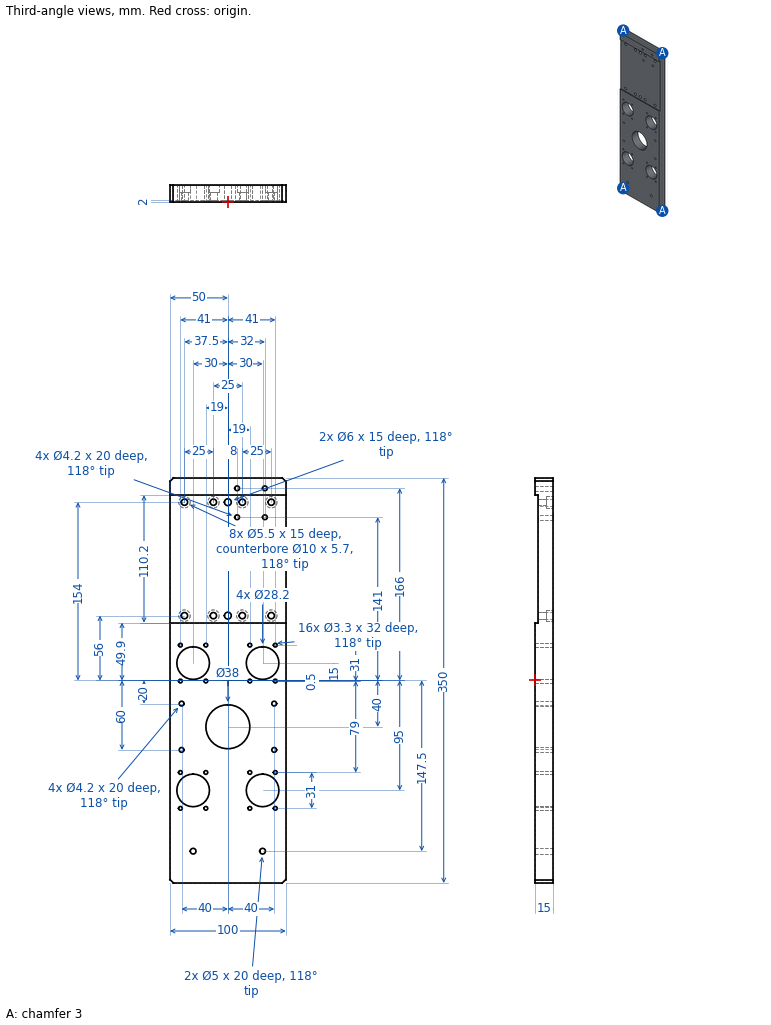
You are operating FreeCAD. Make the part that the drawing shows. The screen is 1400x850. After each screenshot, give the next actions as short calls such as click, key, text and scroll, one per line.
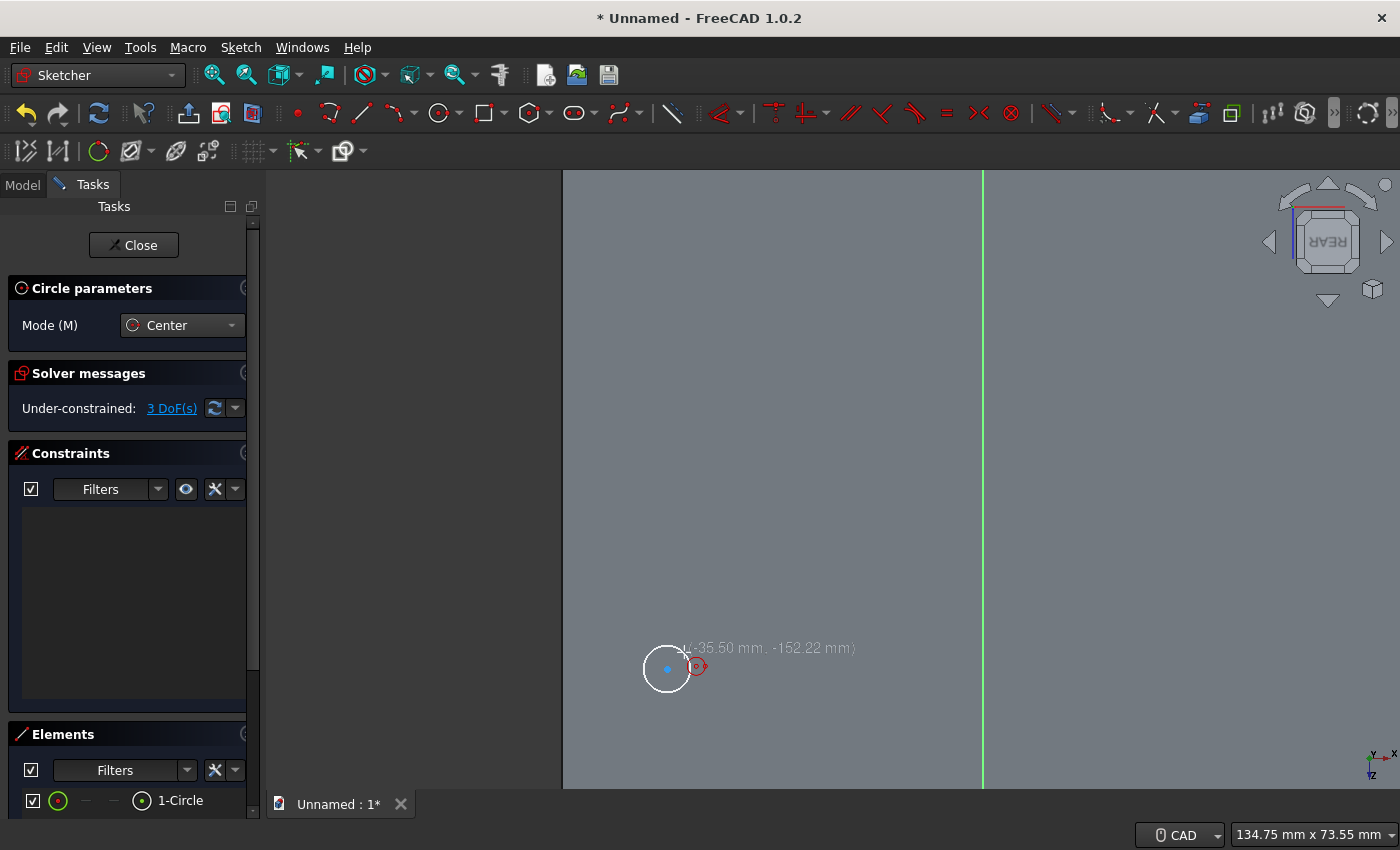
click(878, 668)
click(894, 652)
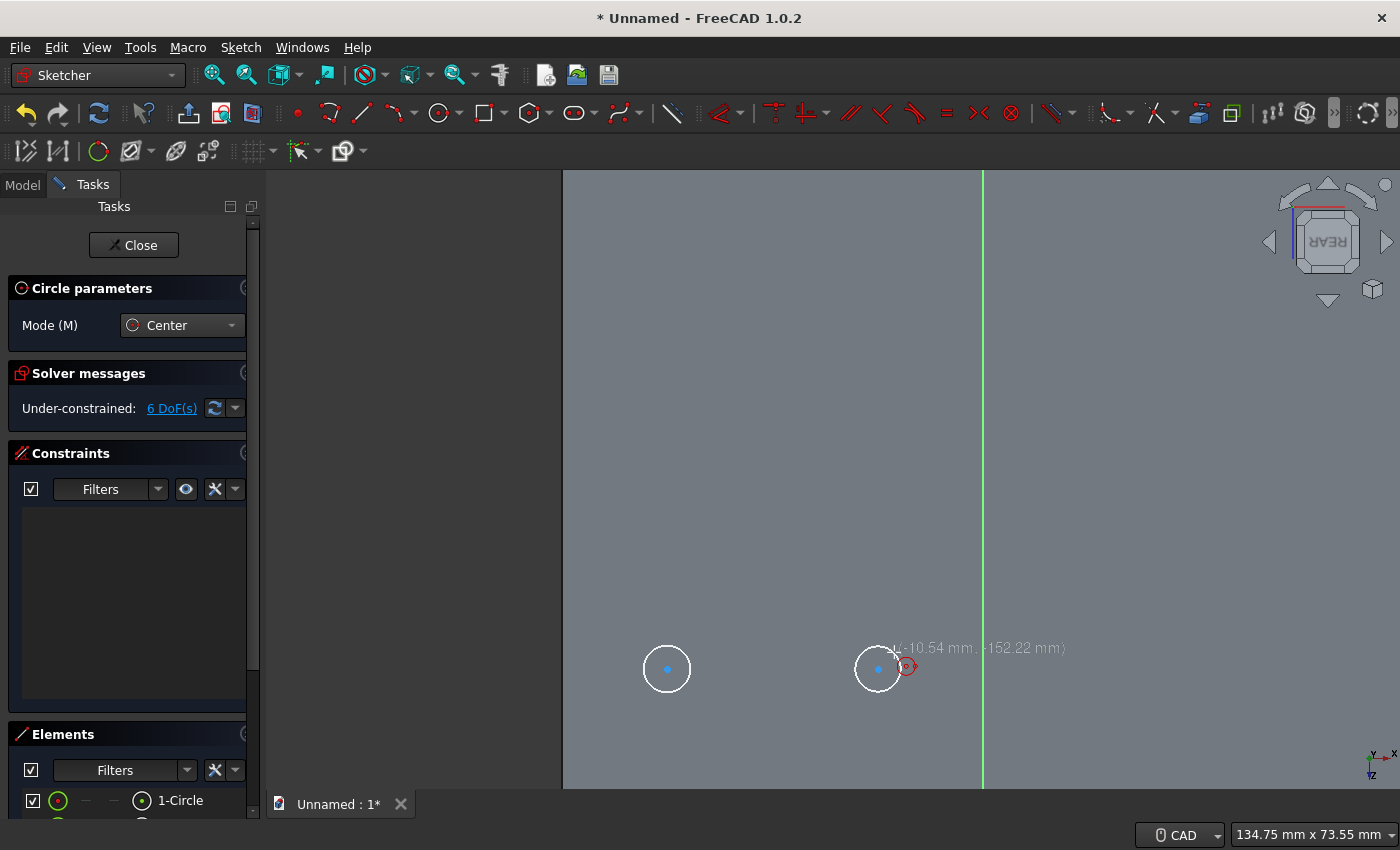
click(1088, 668)
click(1104, 652)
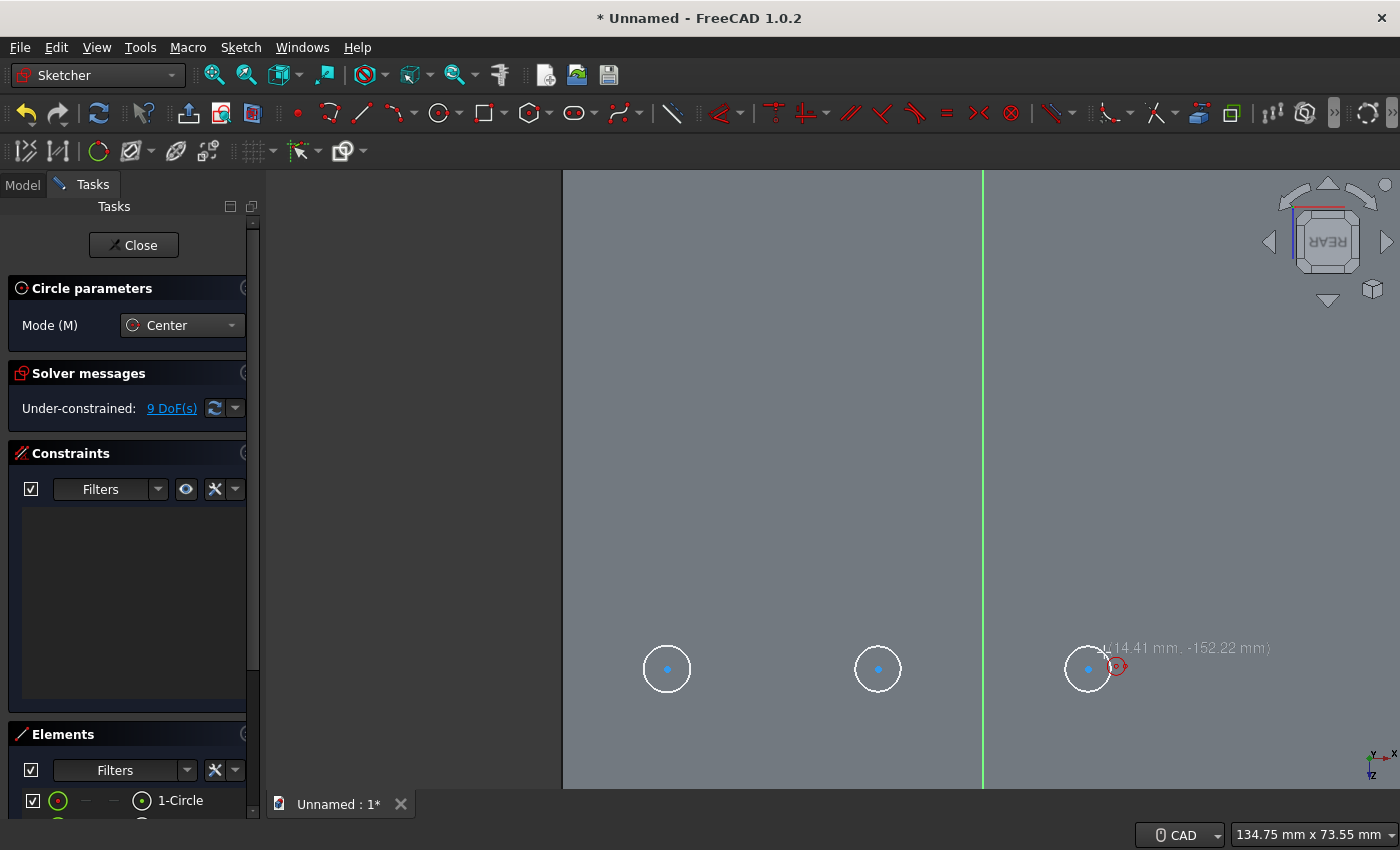
scroll(670, 673, down, 6)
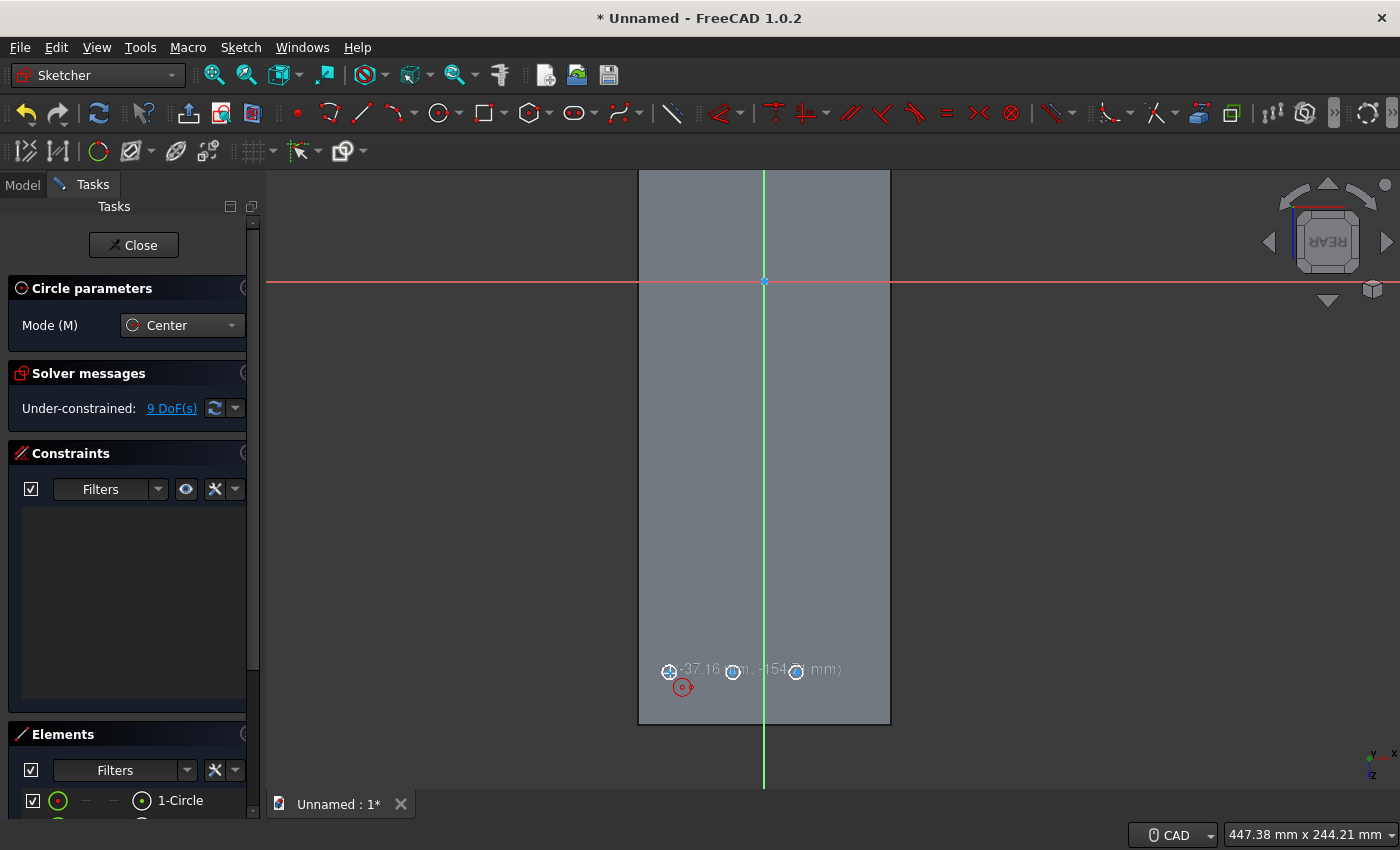
scroll(859, 672, up, 6)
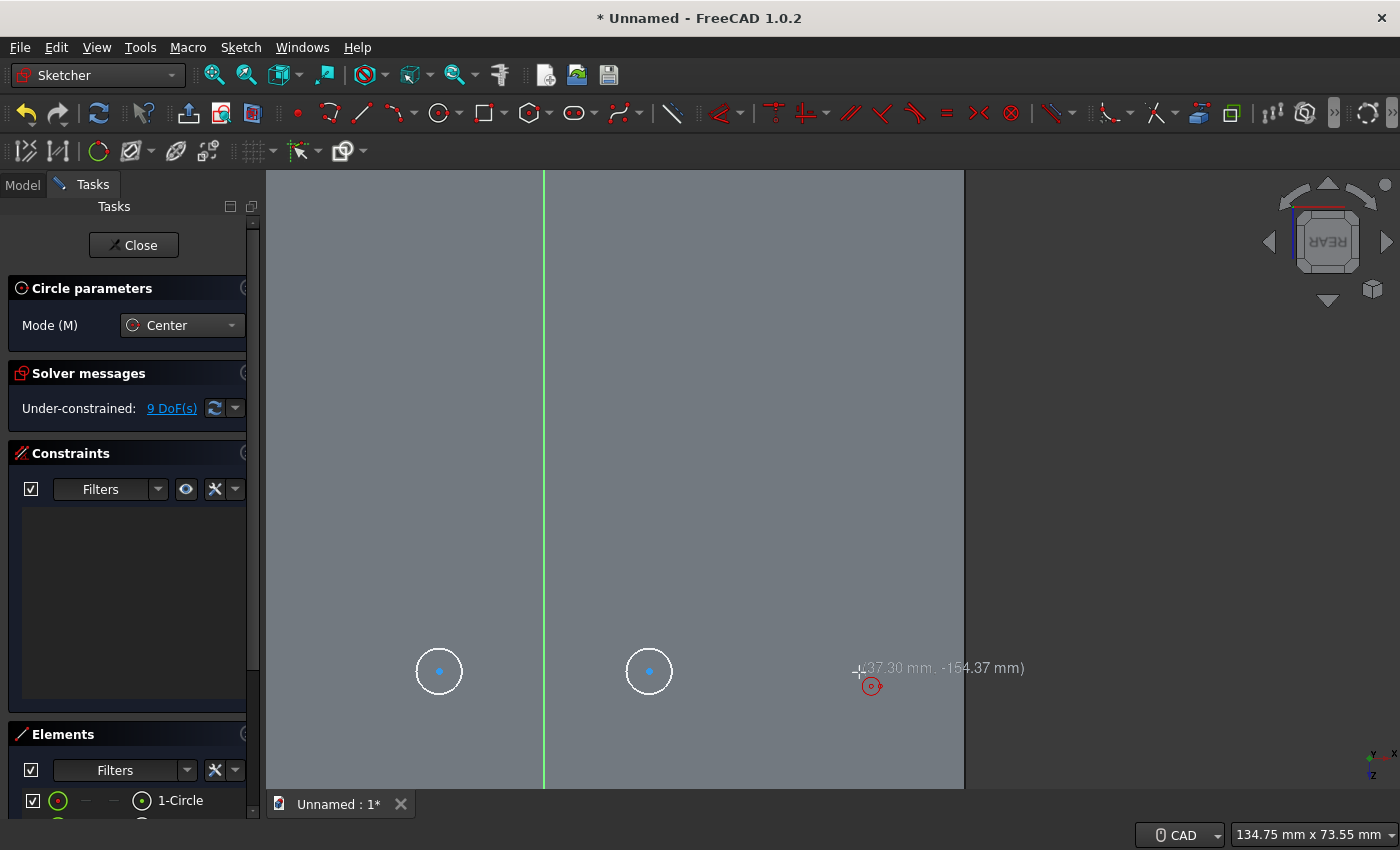
click(859, 670)
click(876, 654)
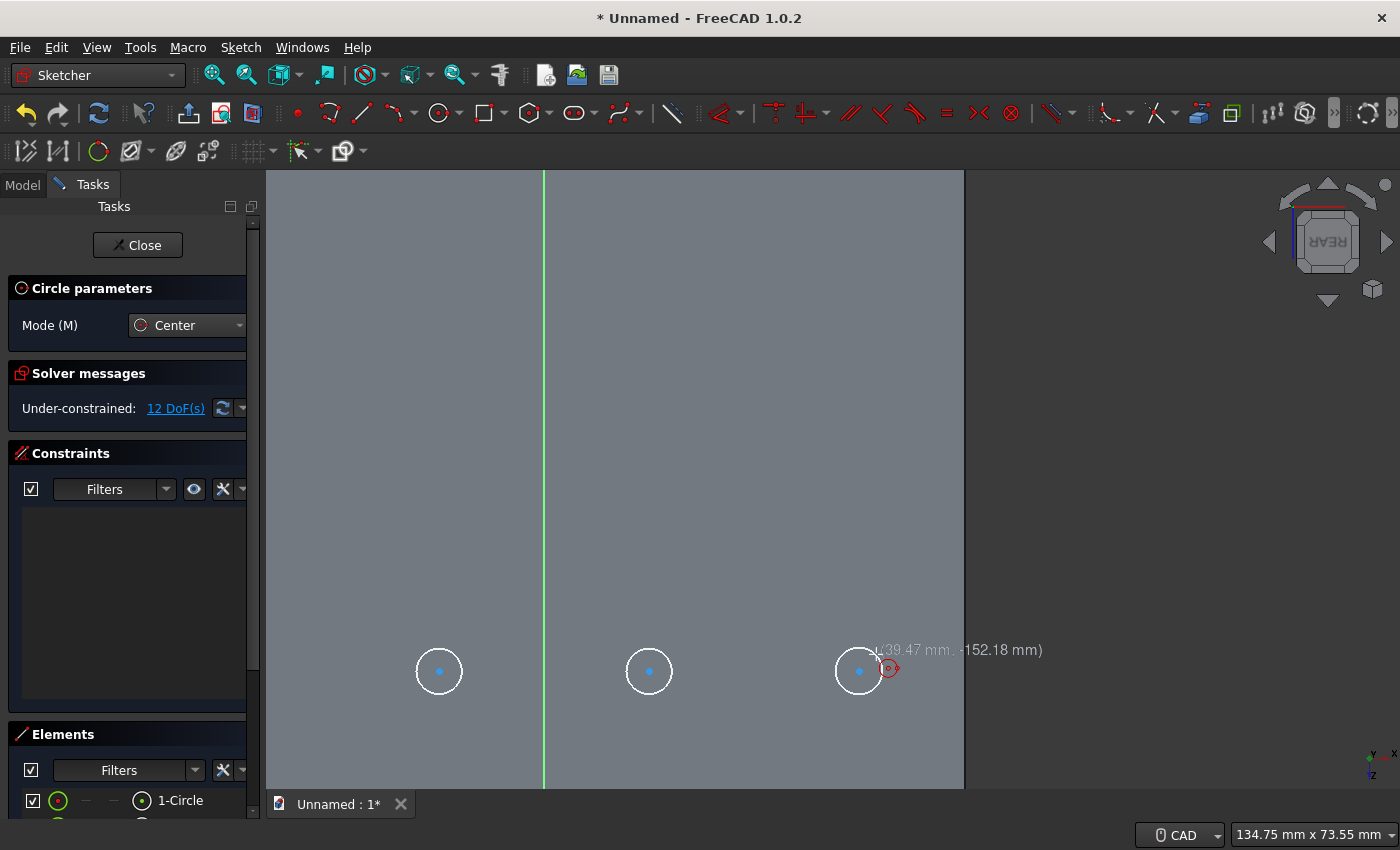
scroll(860, 672, down, 6)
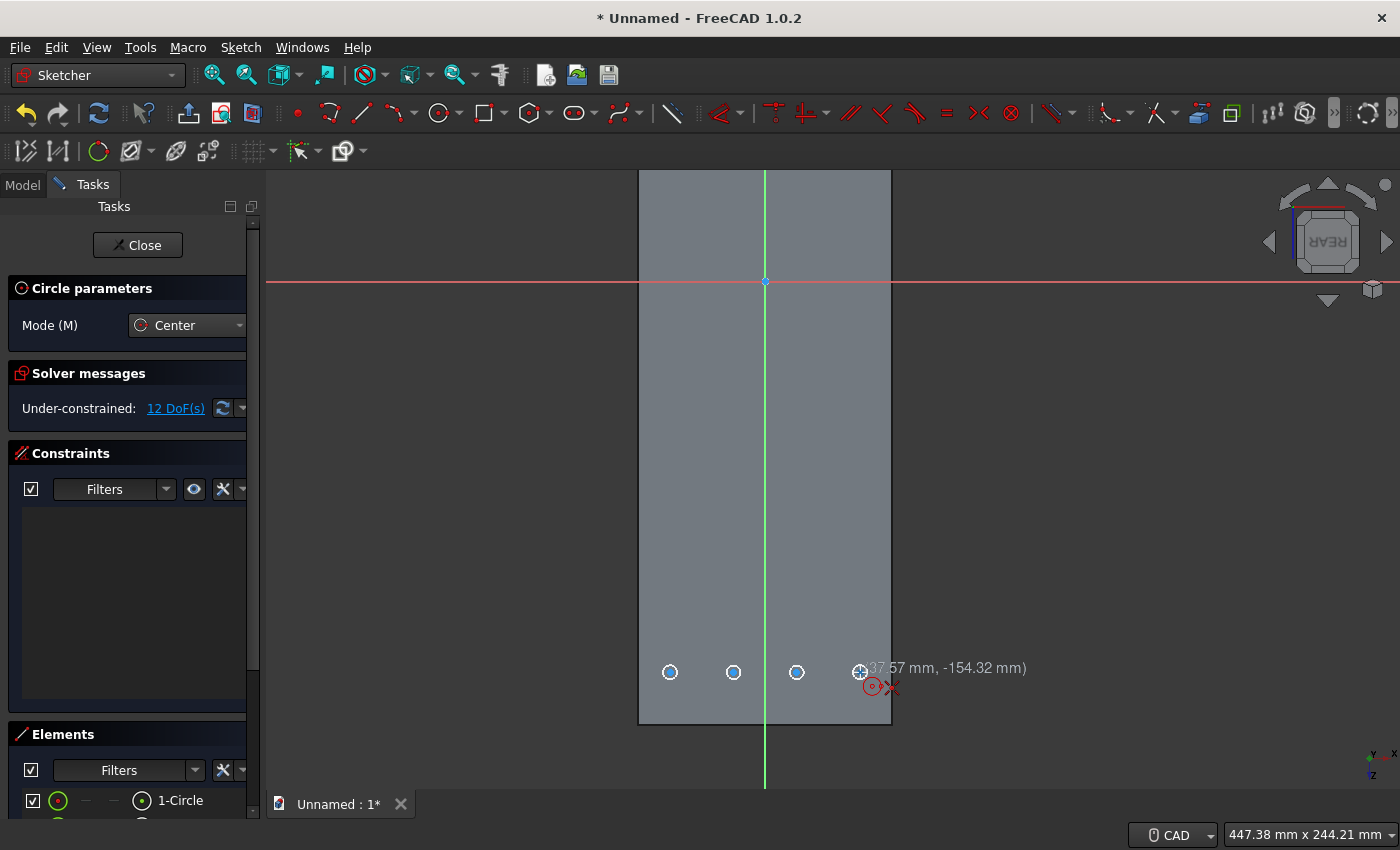
scroll(670, 424, up, 6)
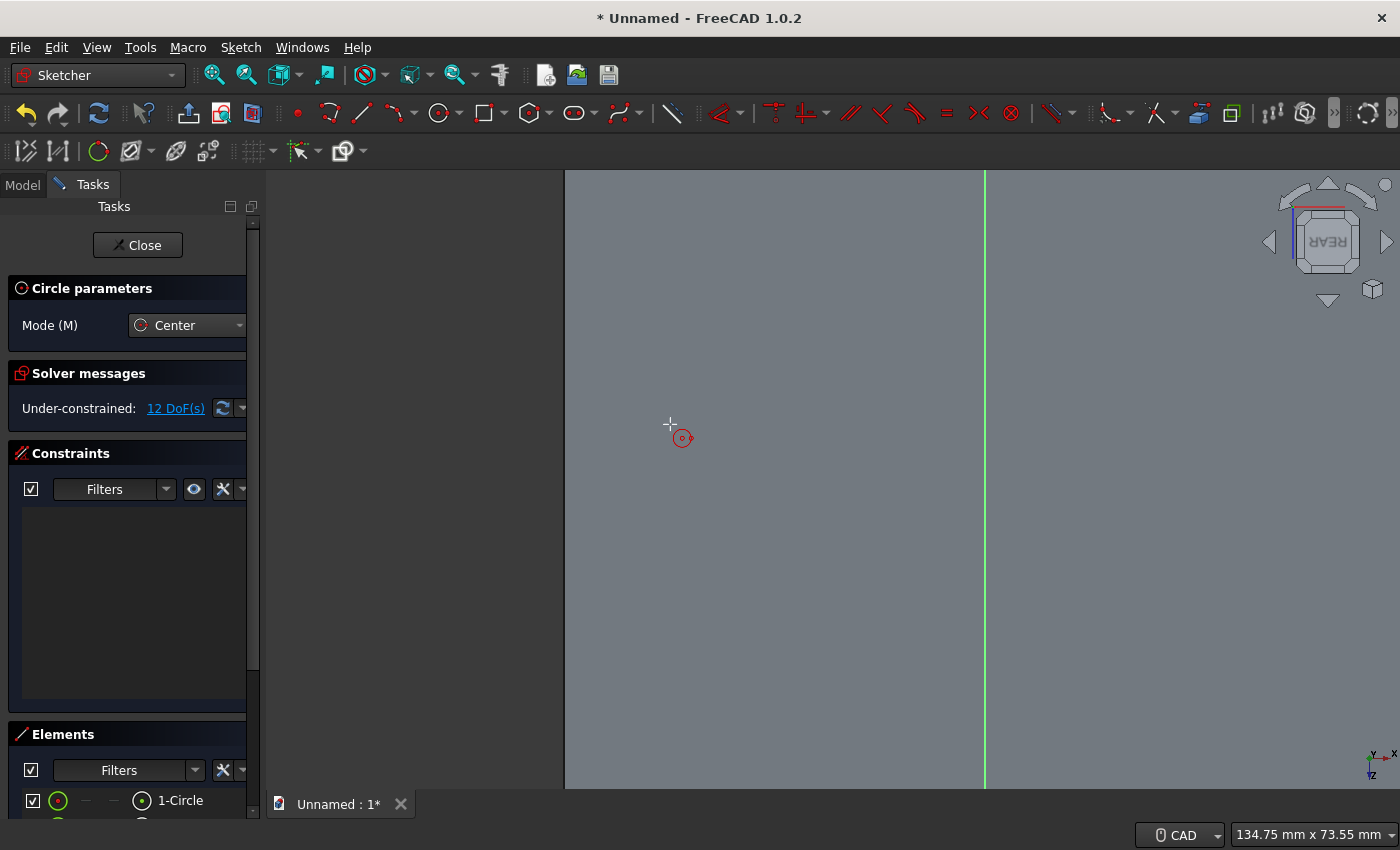
click(669, 422)
click(686, 406)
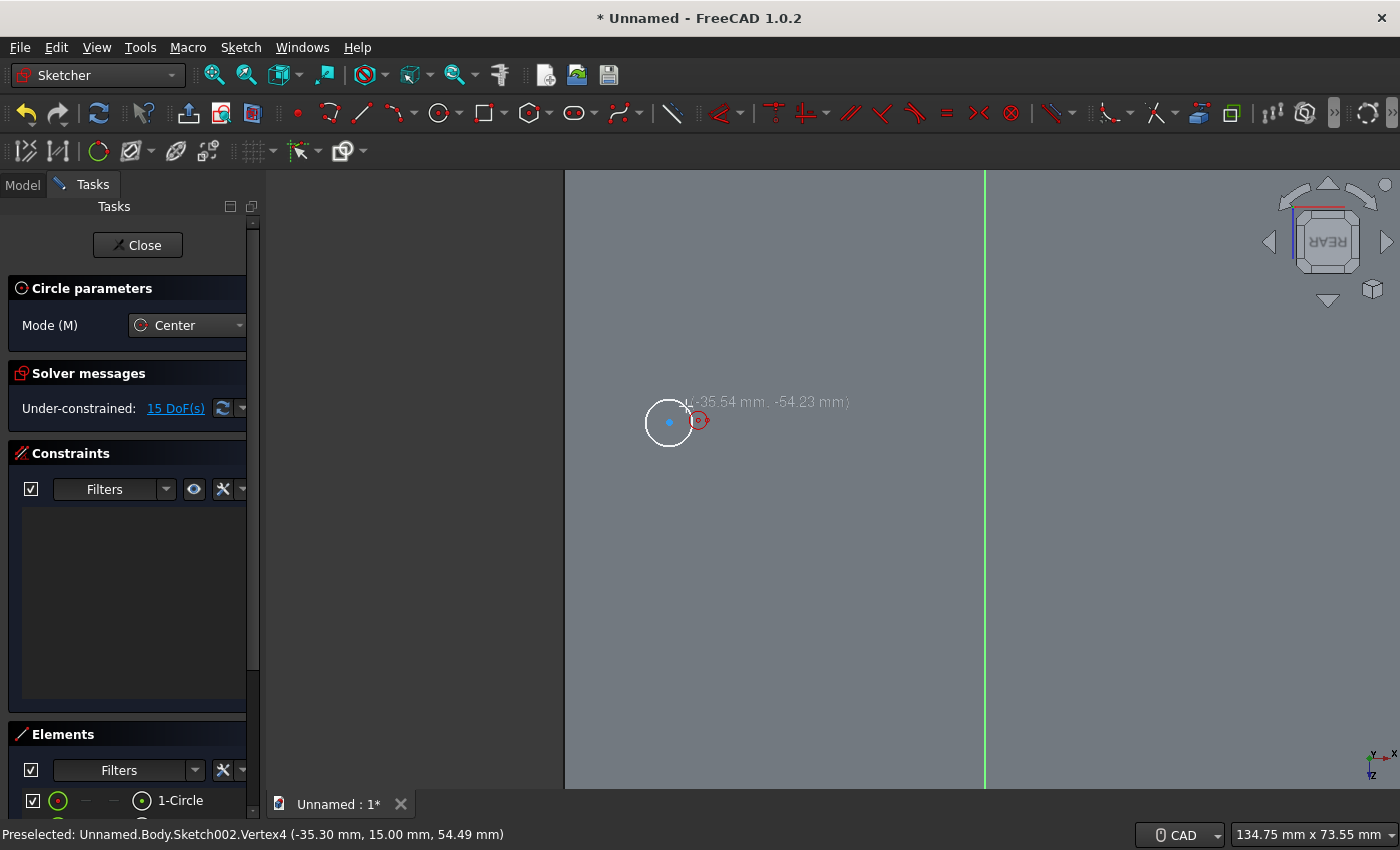
click(880, 422)
click(896, 406)